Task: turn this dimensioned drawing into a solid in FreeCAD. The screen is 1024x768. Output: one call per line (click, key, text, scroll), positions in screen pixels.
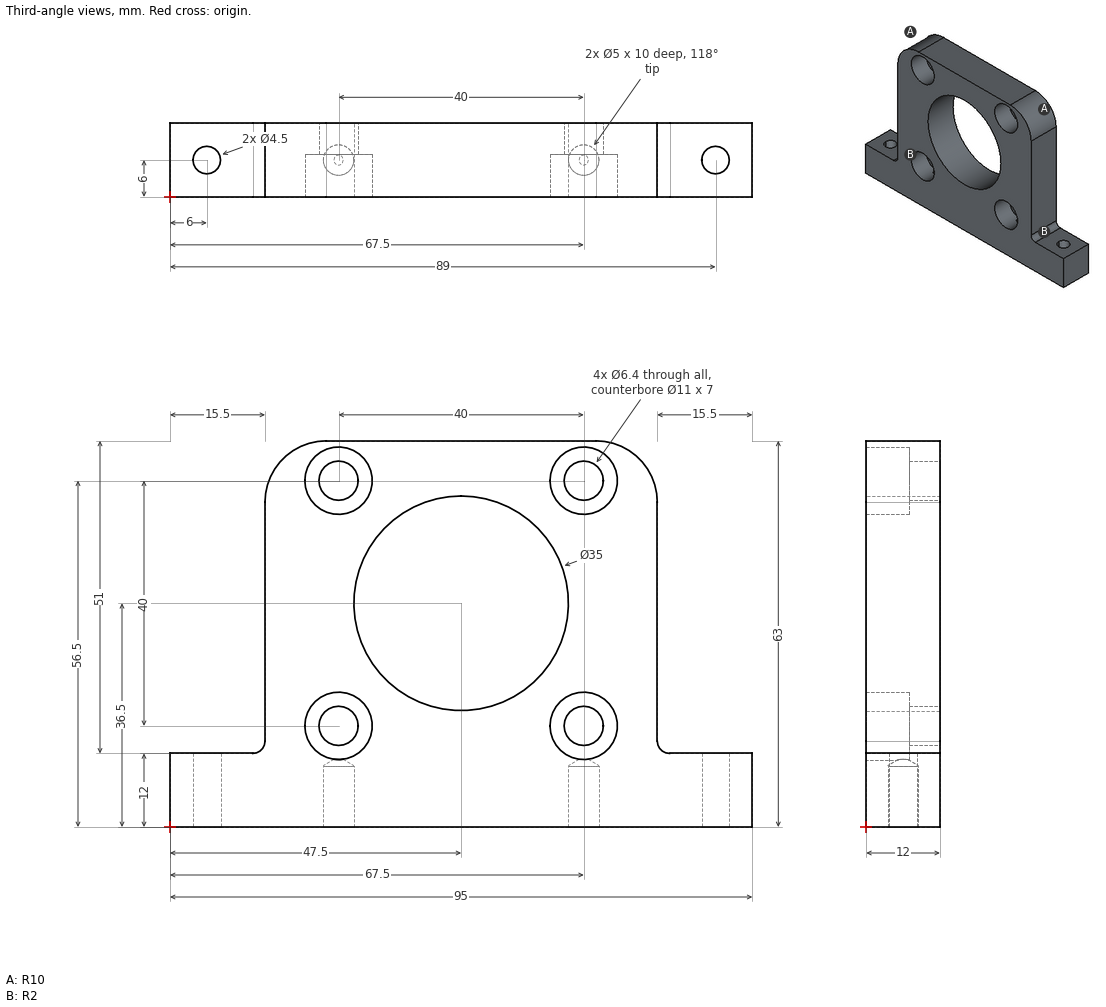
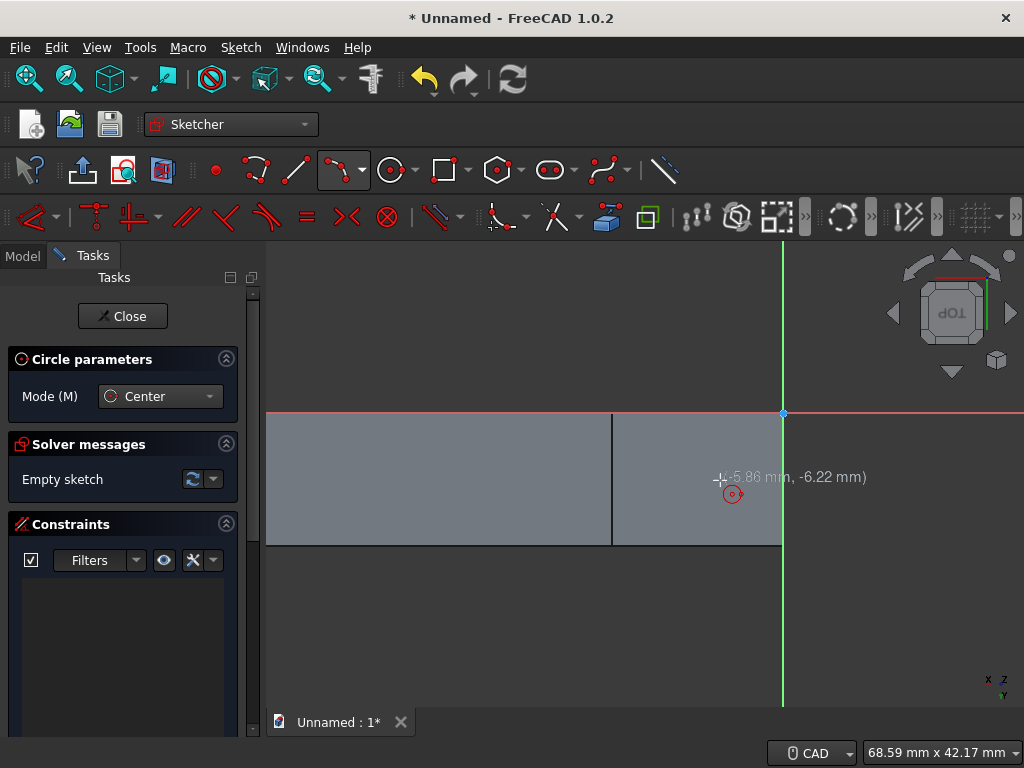
click(717, 480)
click(735, 462)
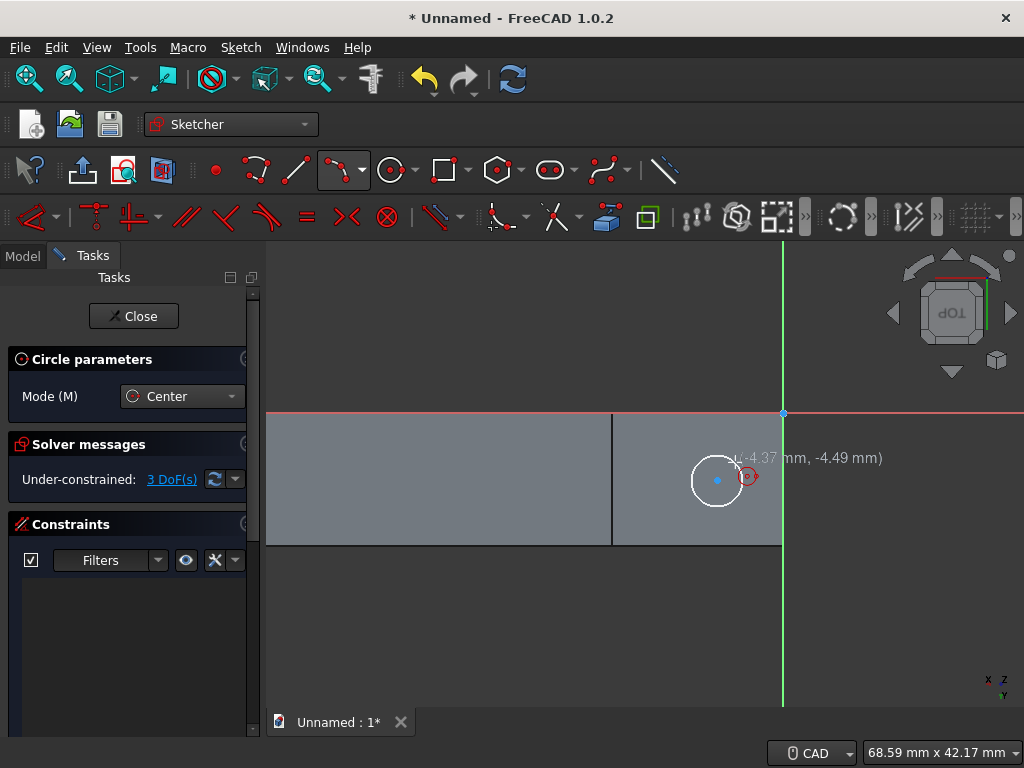
scroll(750, 483, down, 5)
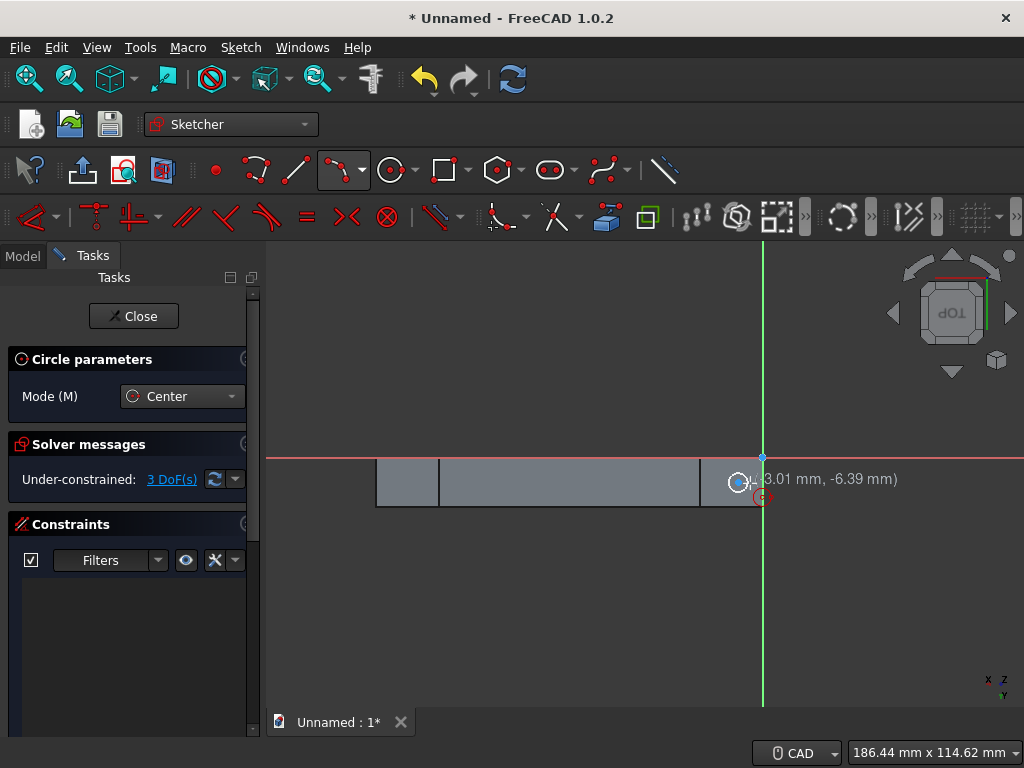
scroll(401, 482, up, 5)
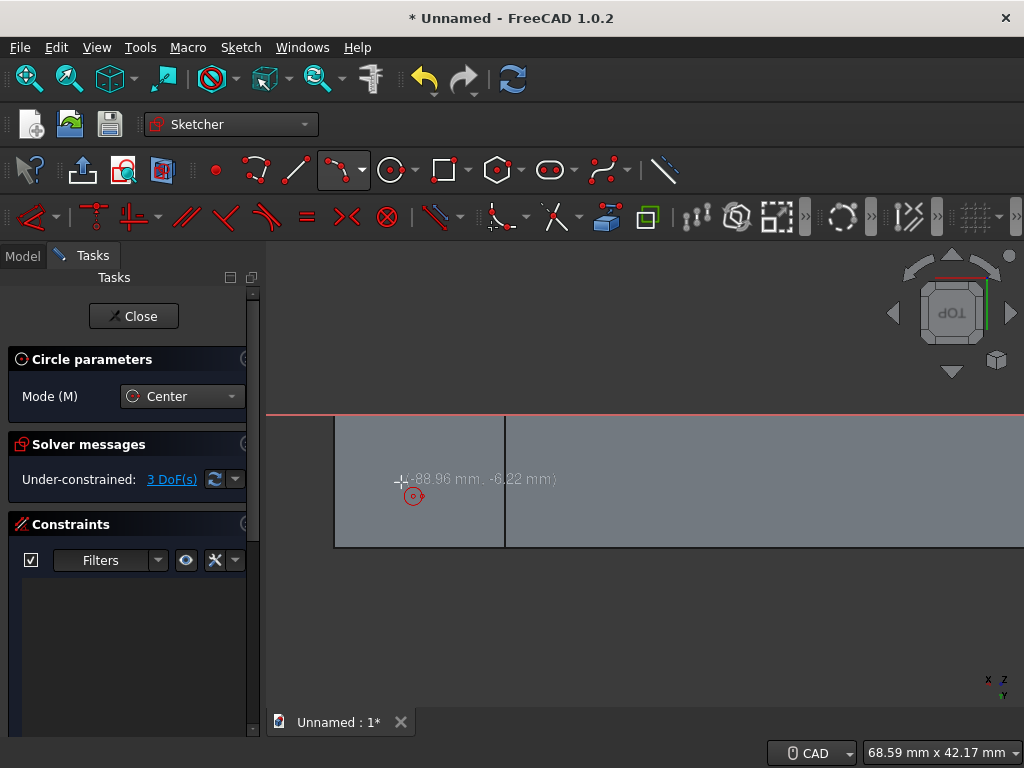
click(400, 481)
click(418, 464)
key(Escape)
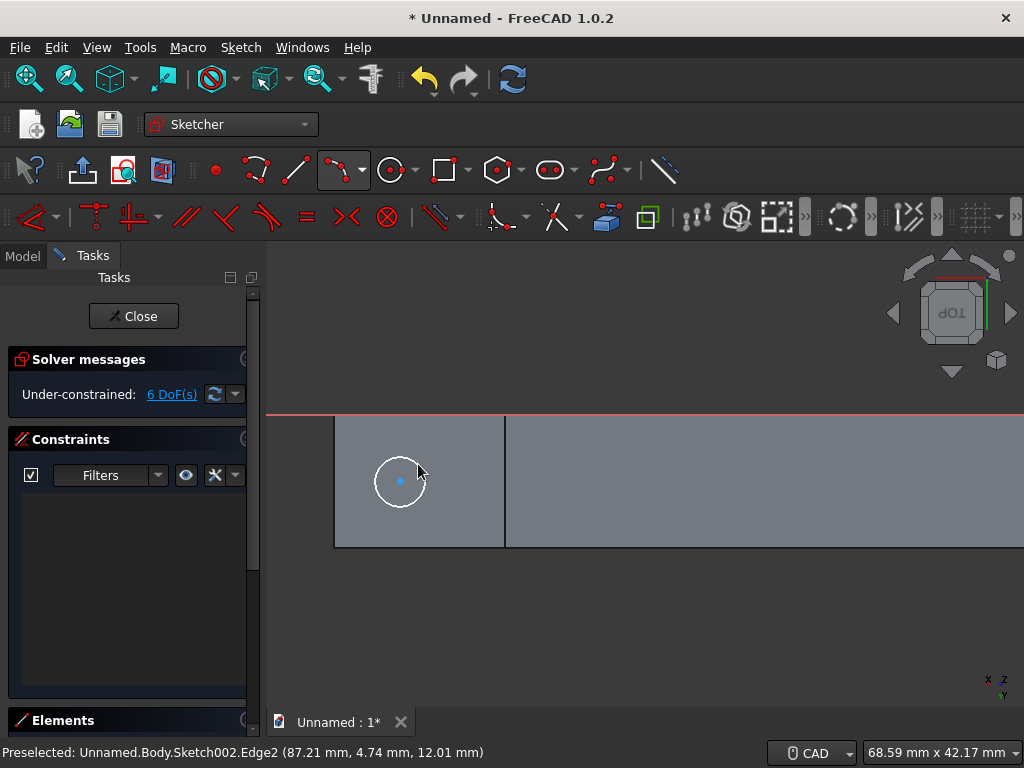
scroll(400, 482, down, 5)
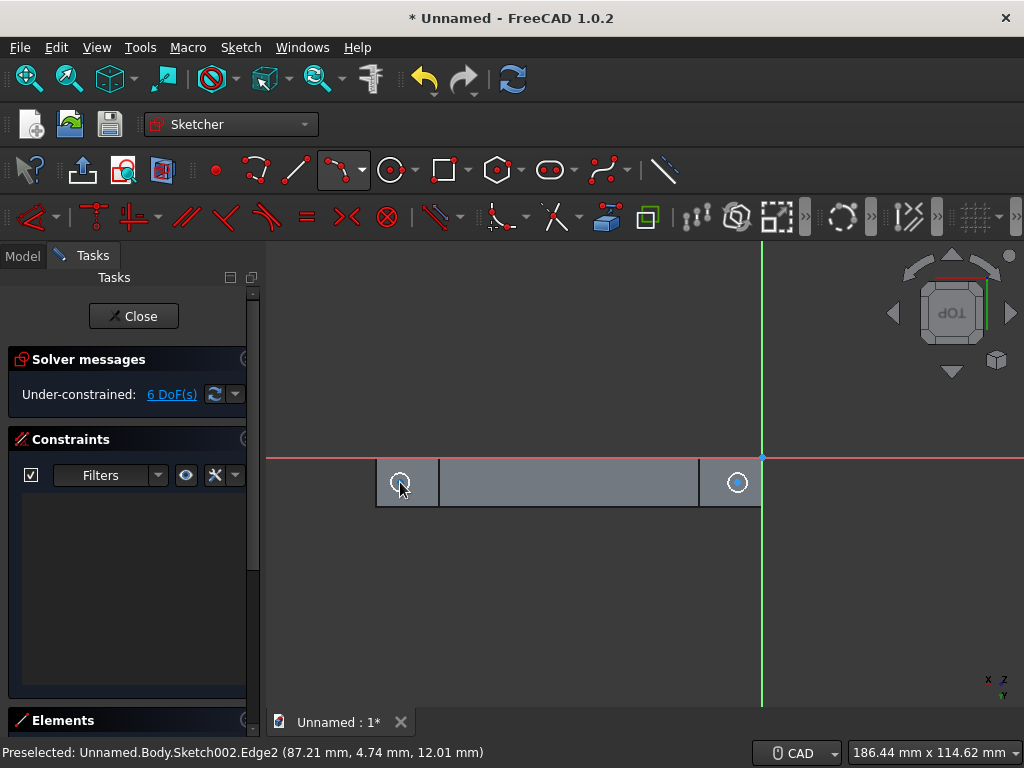
scroll(744, 476, up, 2)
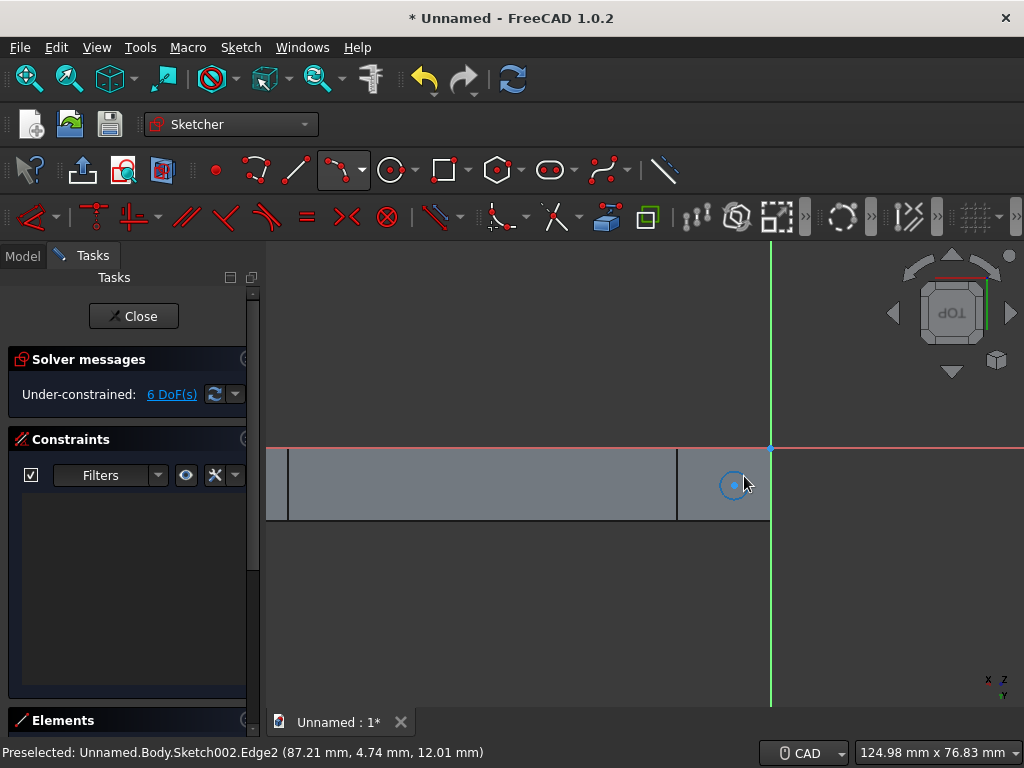
click(744, 476)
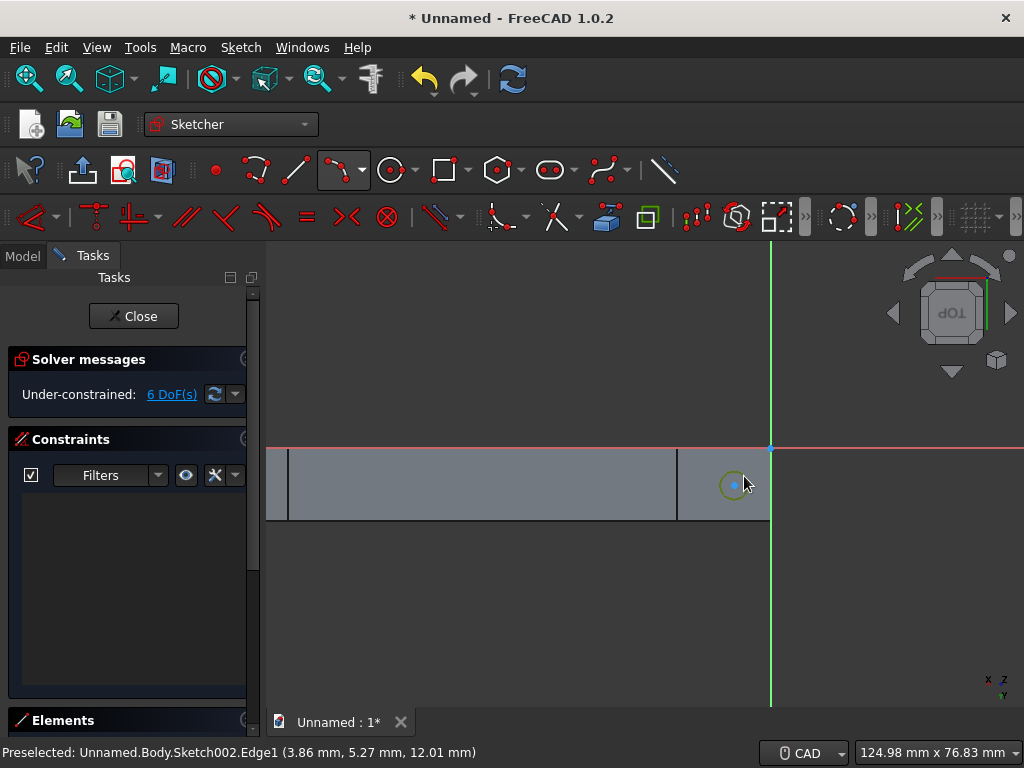
scroll(745, 475, down, 2)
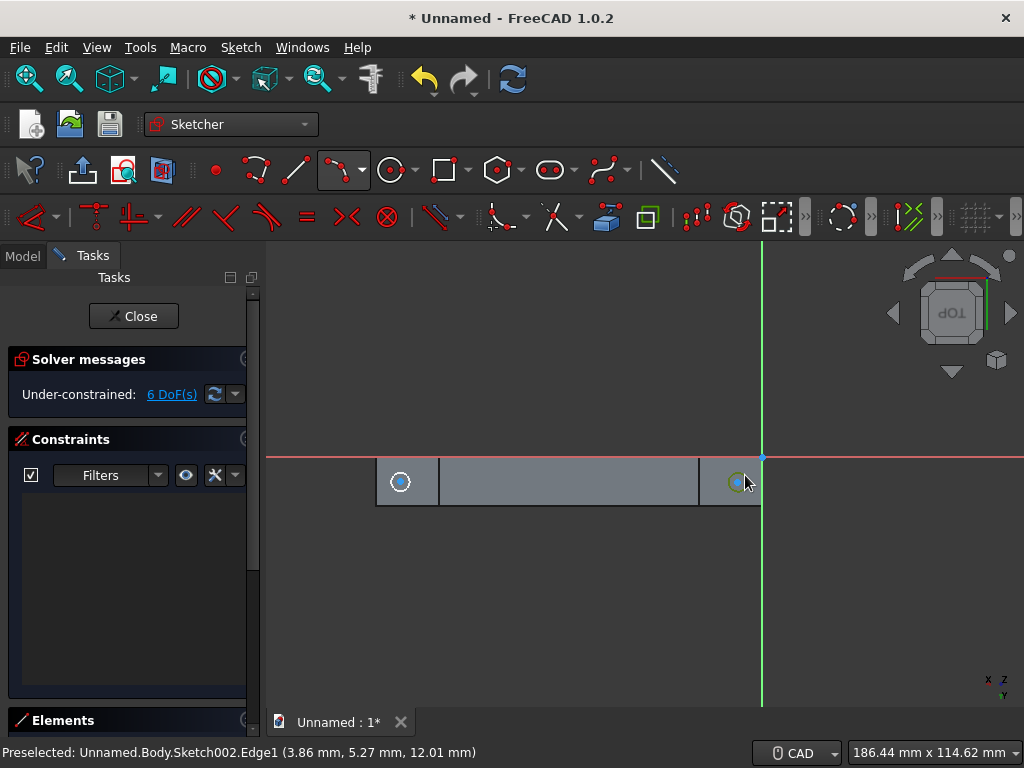
scroll(407, 476, up, 3)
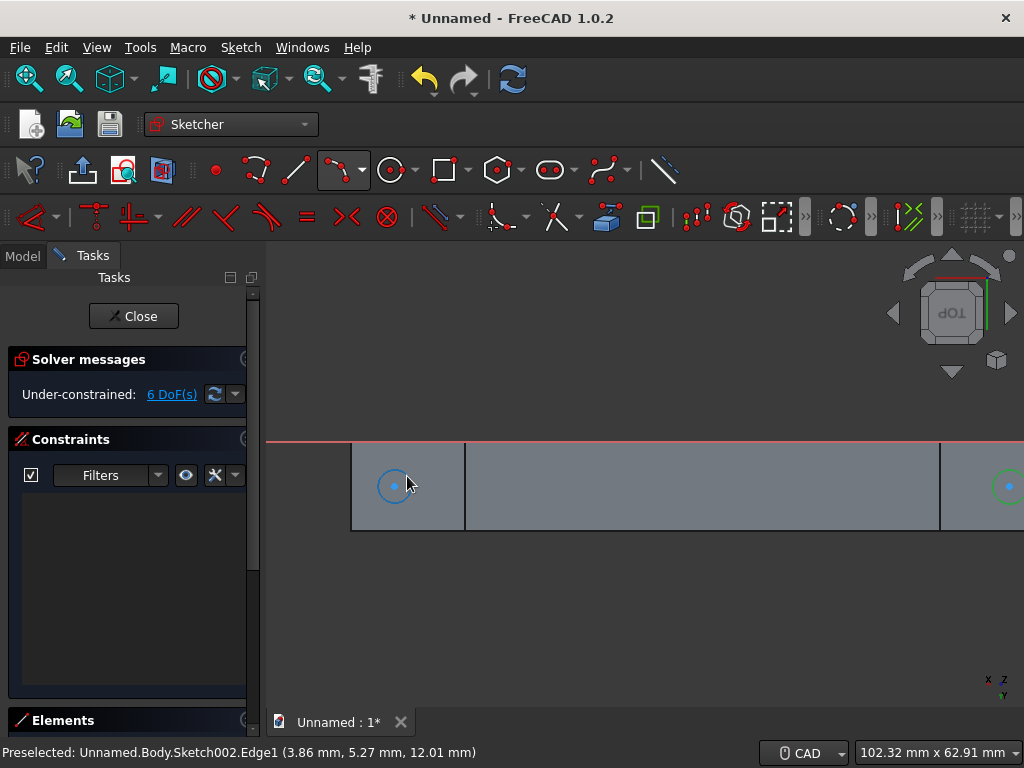
click(407, 475)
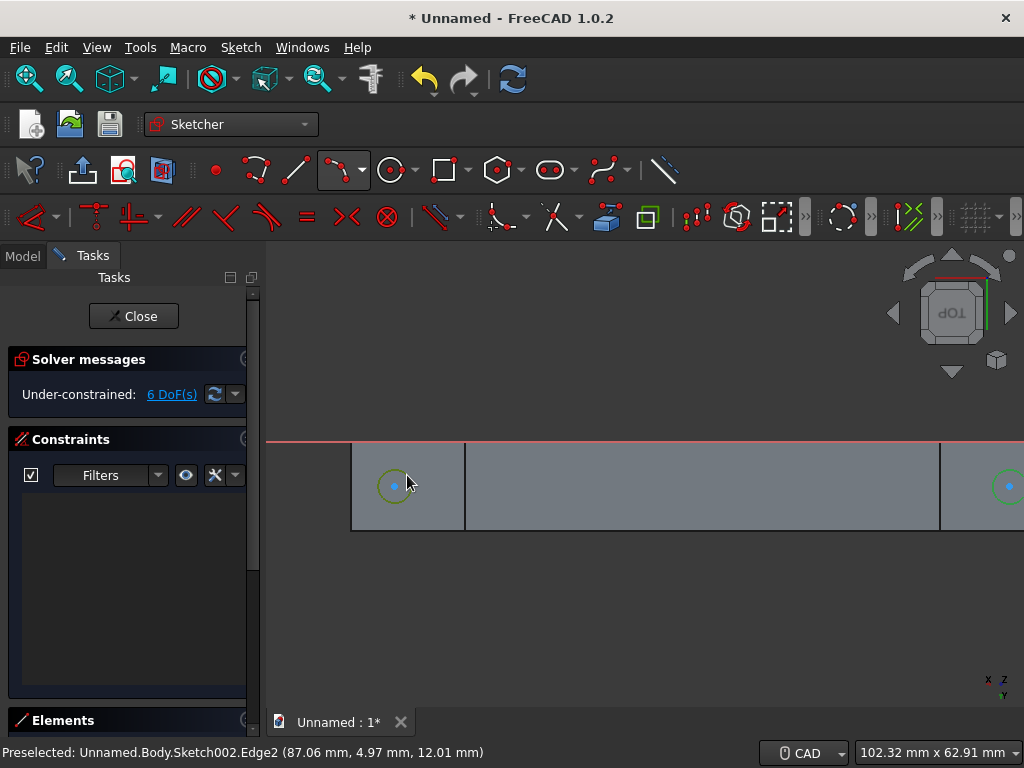
key(e)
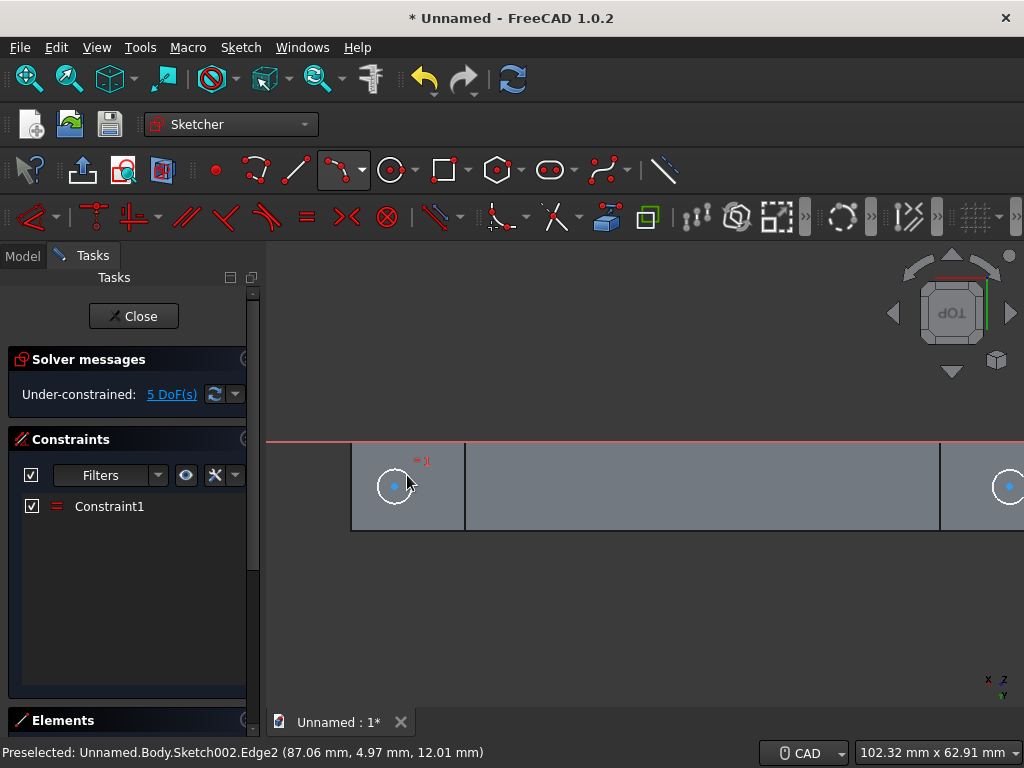
scroll(406, 476, down, 3)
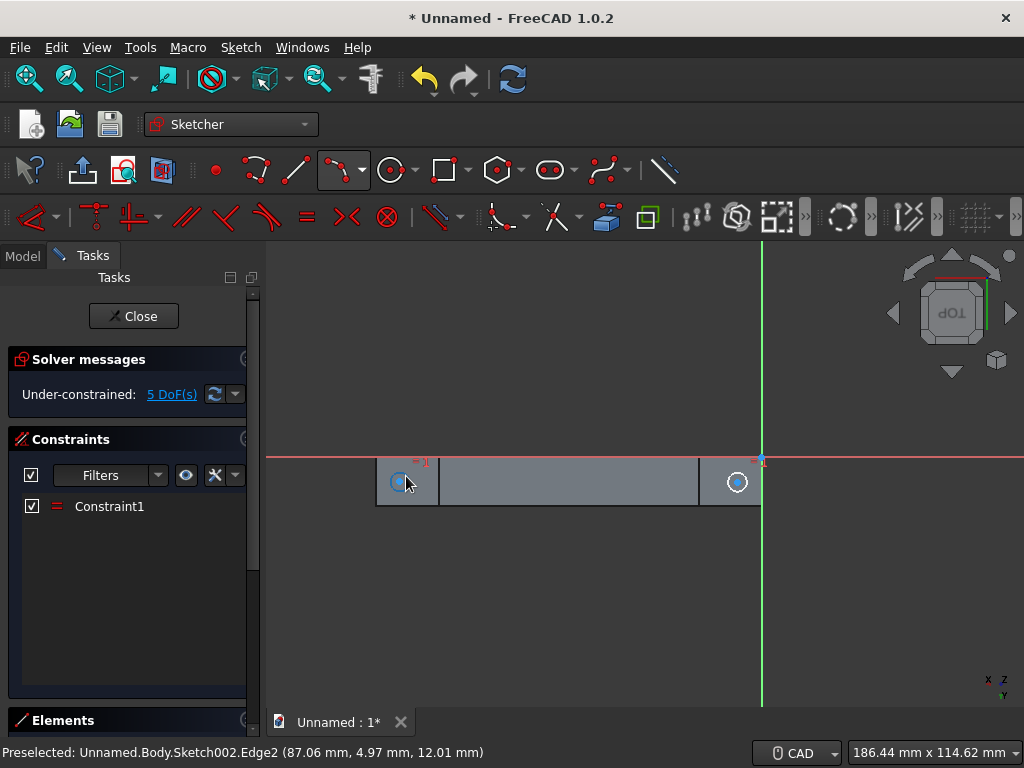
click(738, 482)